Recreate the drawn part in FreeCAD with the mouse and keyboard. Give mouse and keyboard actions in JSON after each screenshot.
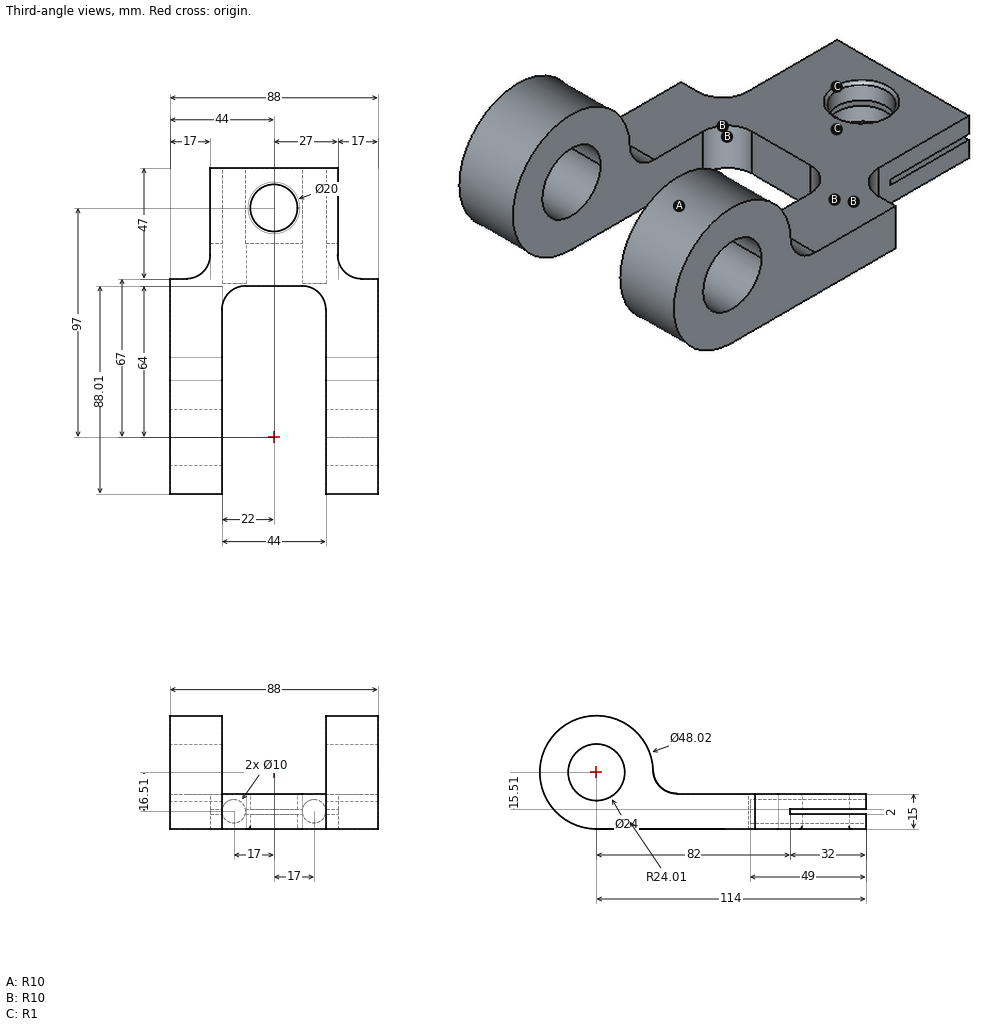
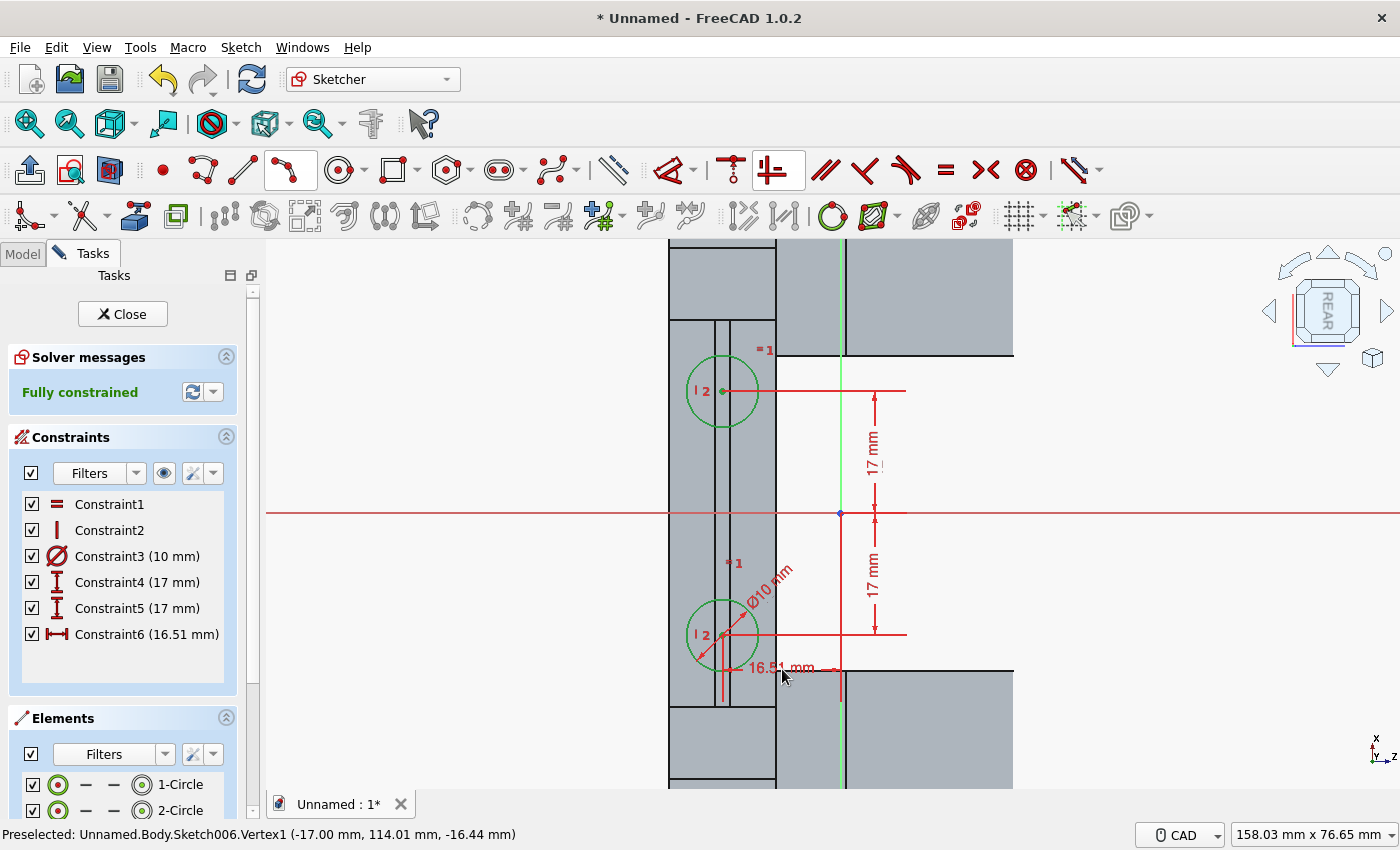
{"action": "left_click", "coordinate": [123, 314]}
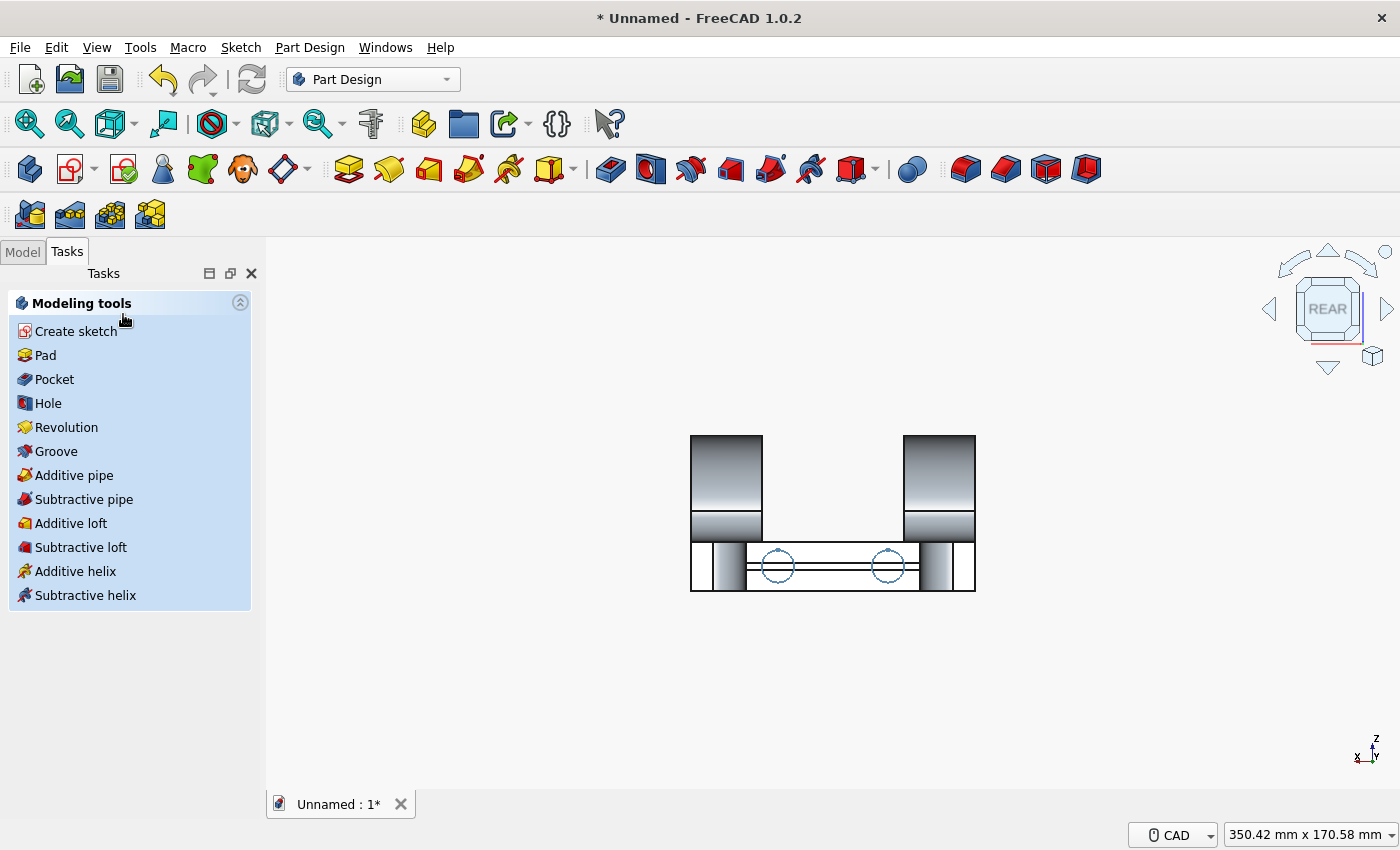
{"action": "left_click", "coordinate": [612, 170]}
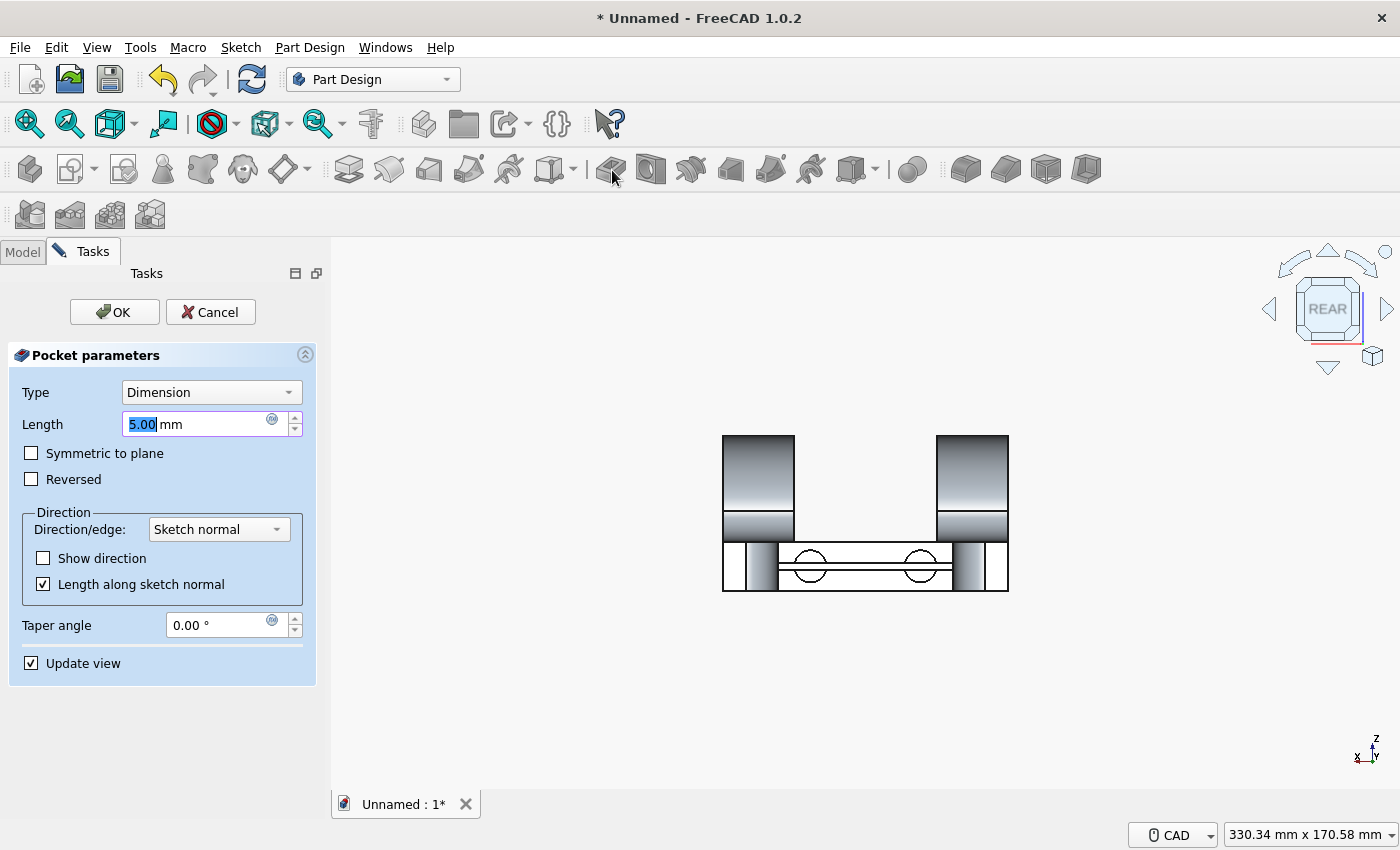
{"action": "type", "text": "49"}
{"action": "key", "text": "Tab"}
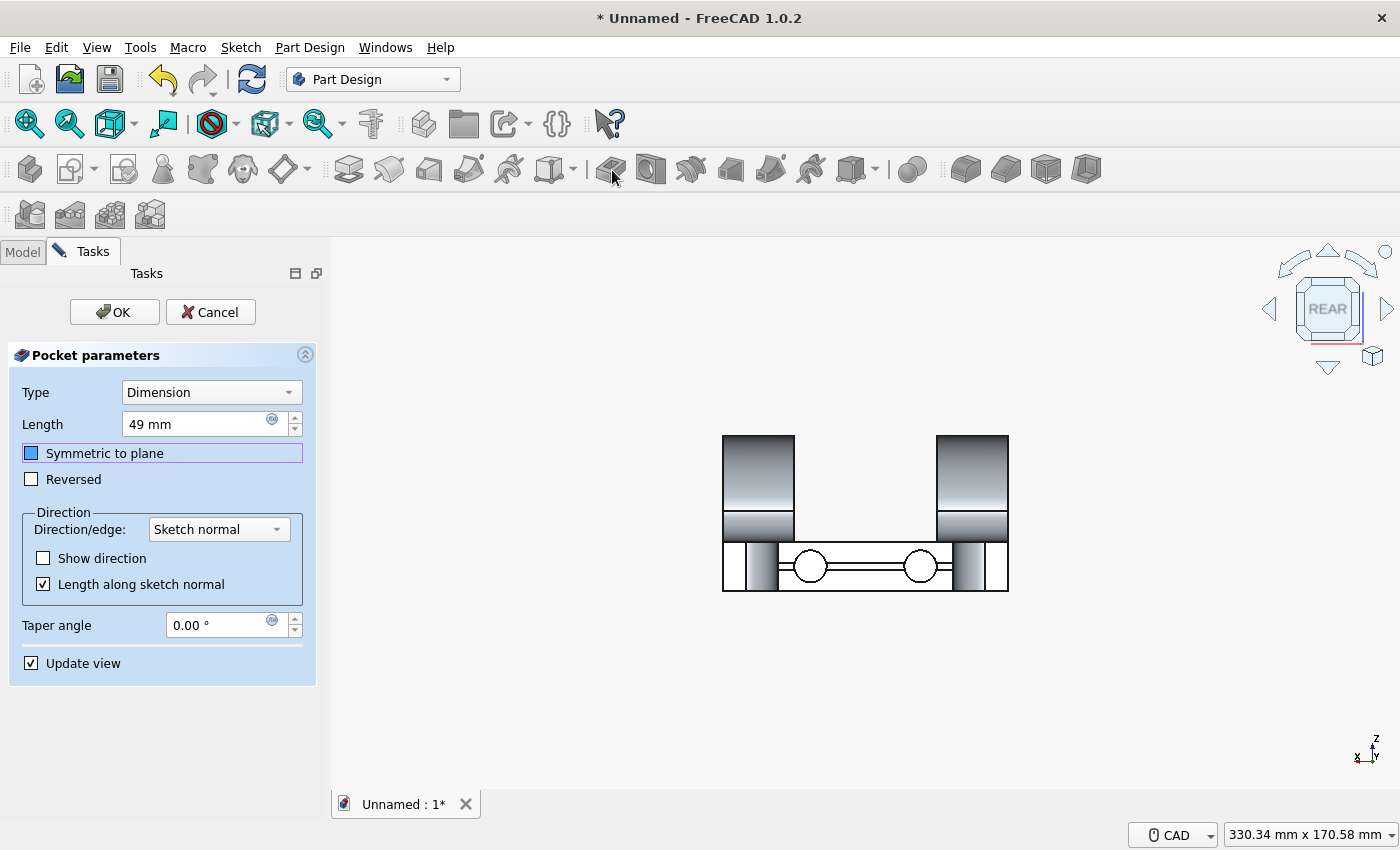
{"action": "left_click", "coordinate": [115, 312]}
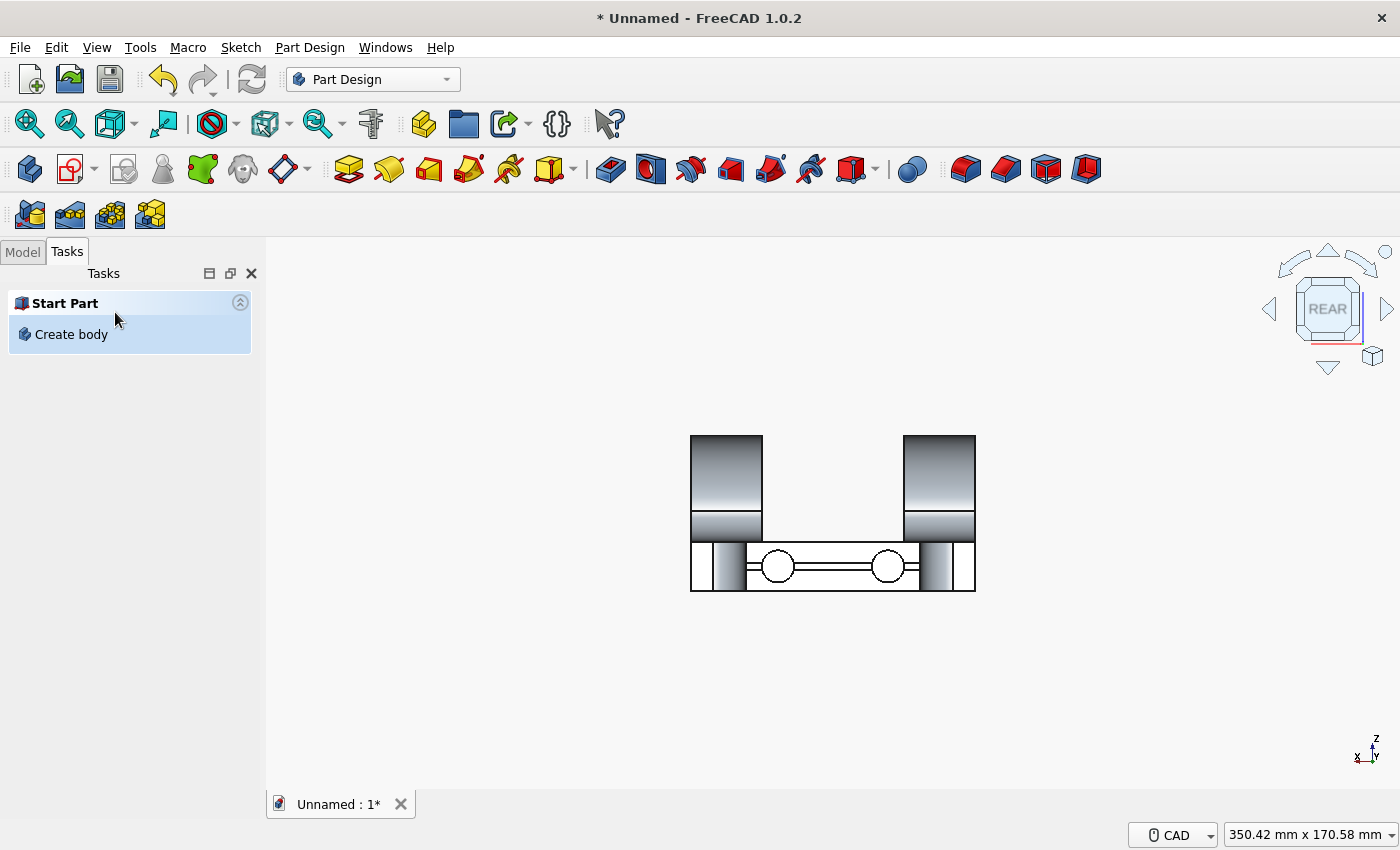
{"action": "key", "text": "0"}